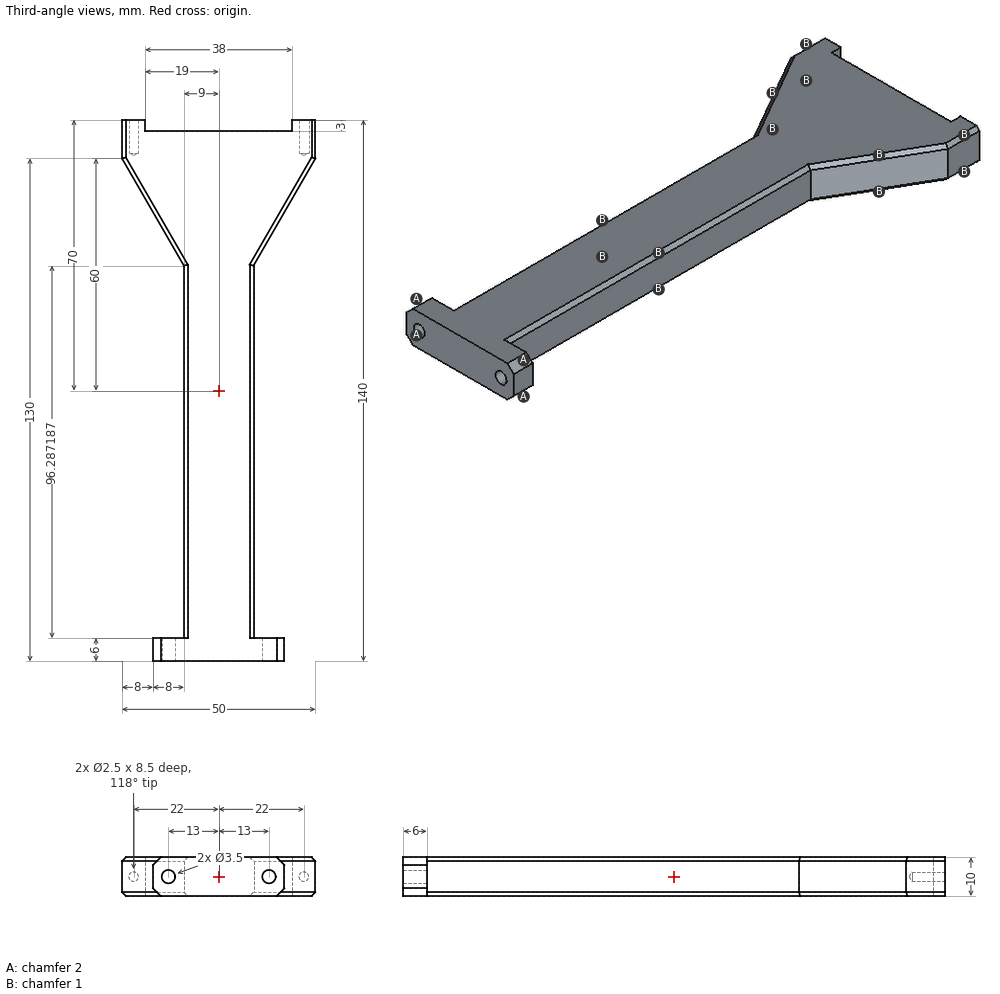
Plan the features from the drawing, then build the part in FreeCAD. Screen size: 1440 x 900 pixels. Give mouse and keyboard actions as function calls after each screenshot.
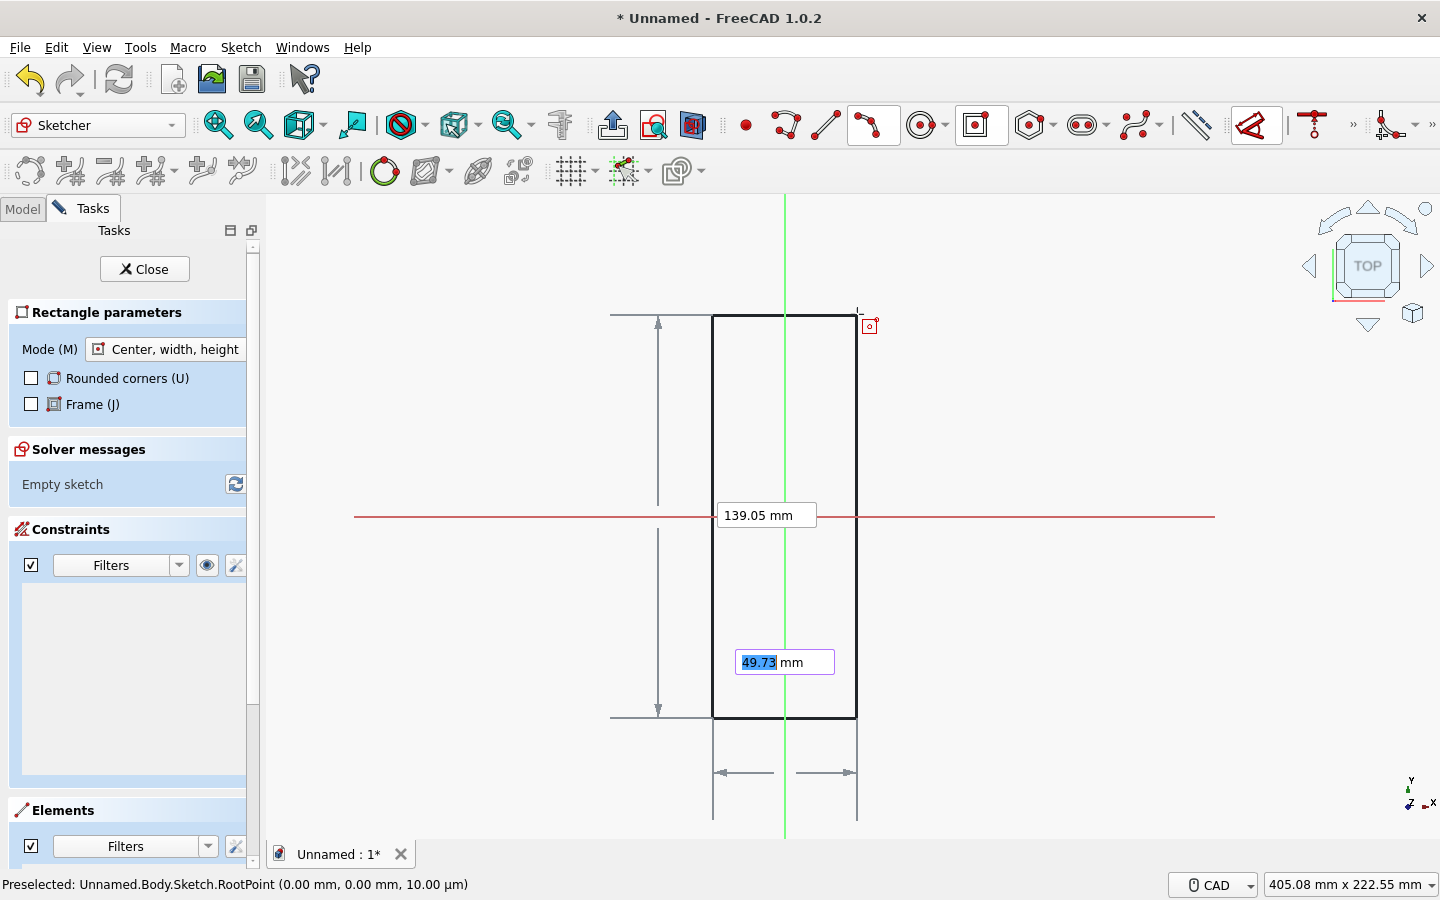
text(50)
key(Tab)
text(140)
key(Return)
key(Escape)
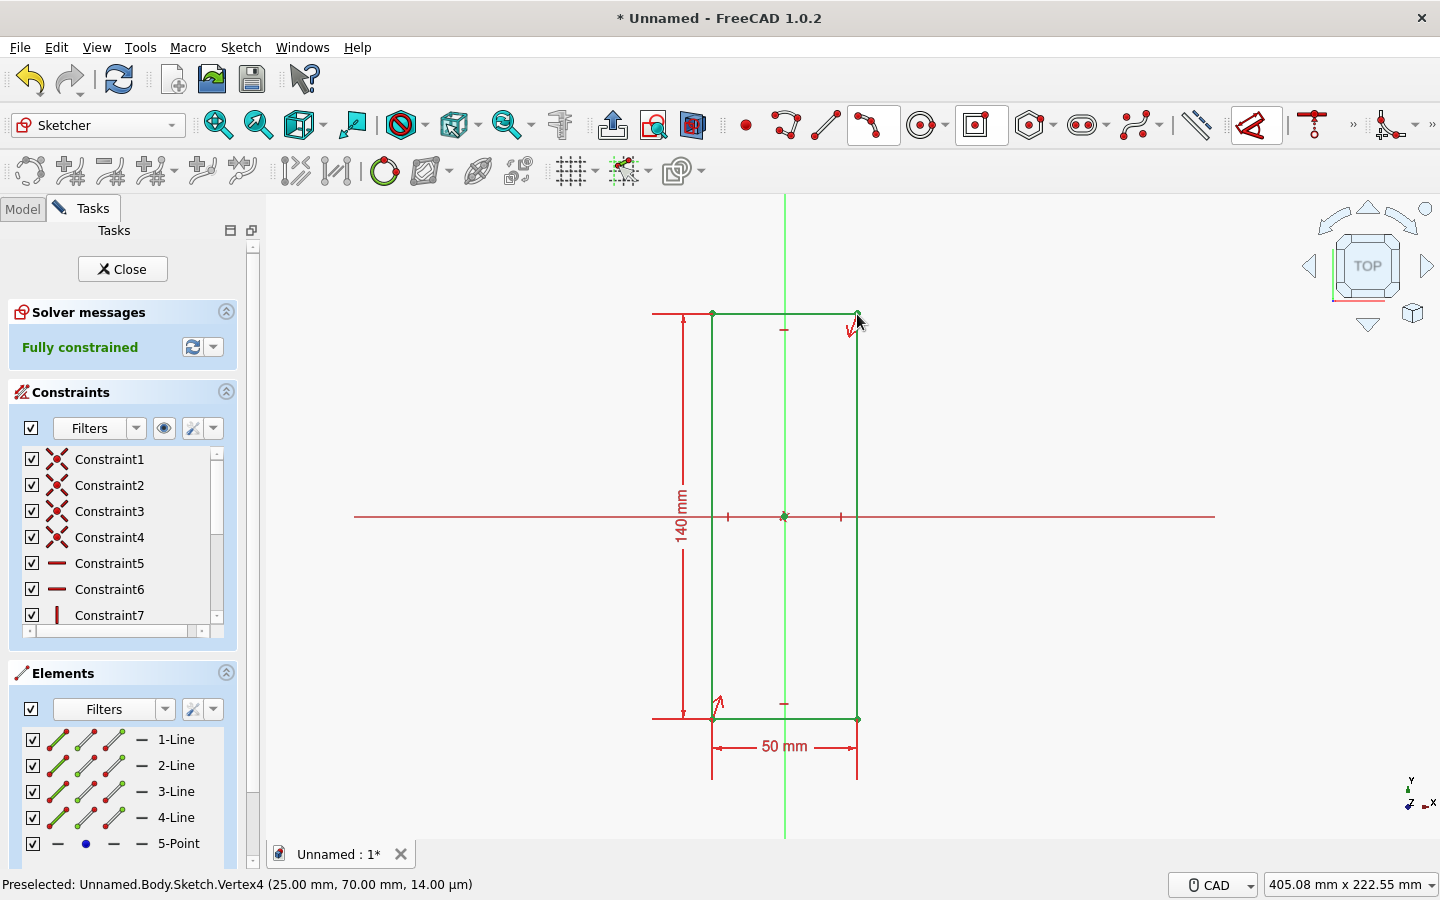
click(123, 269)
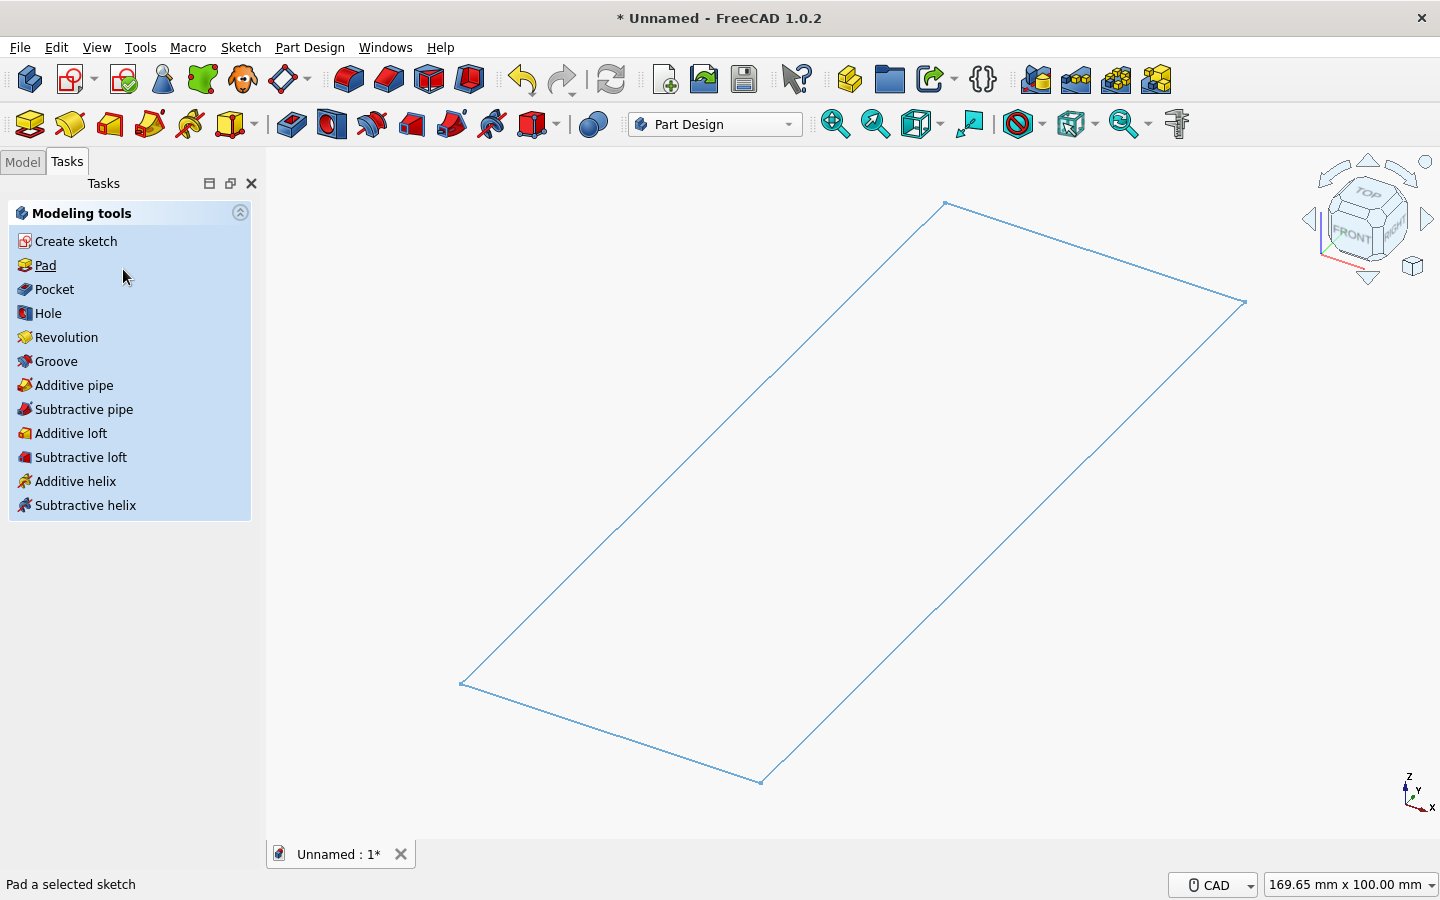
click(30, 124)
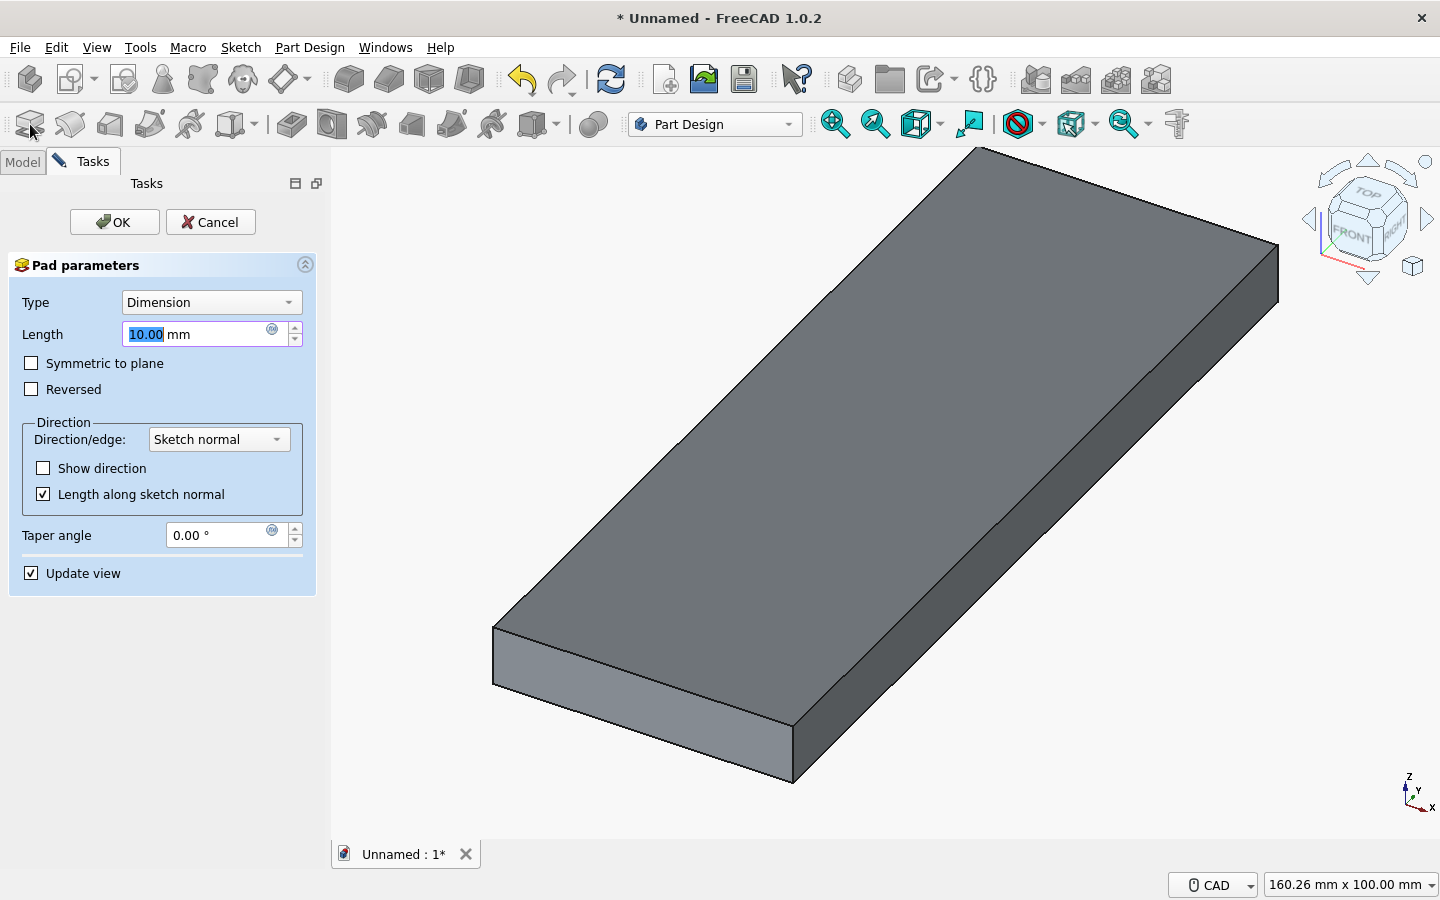
text(10)
key(Tab)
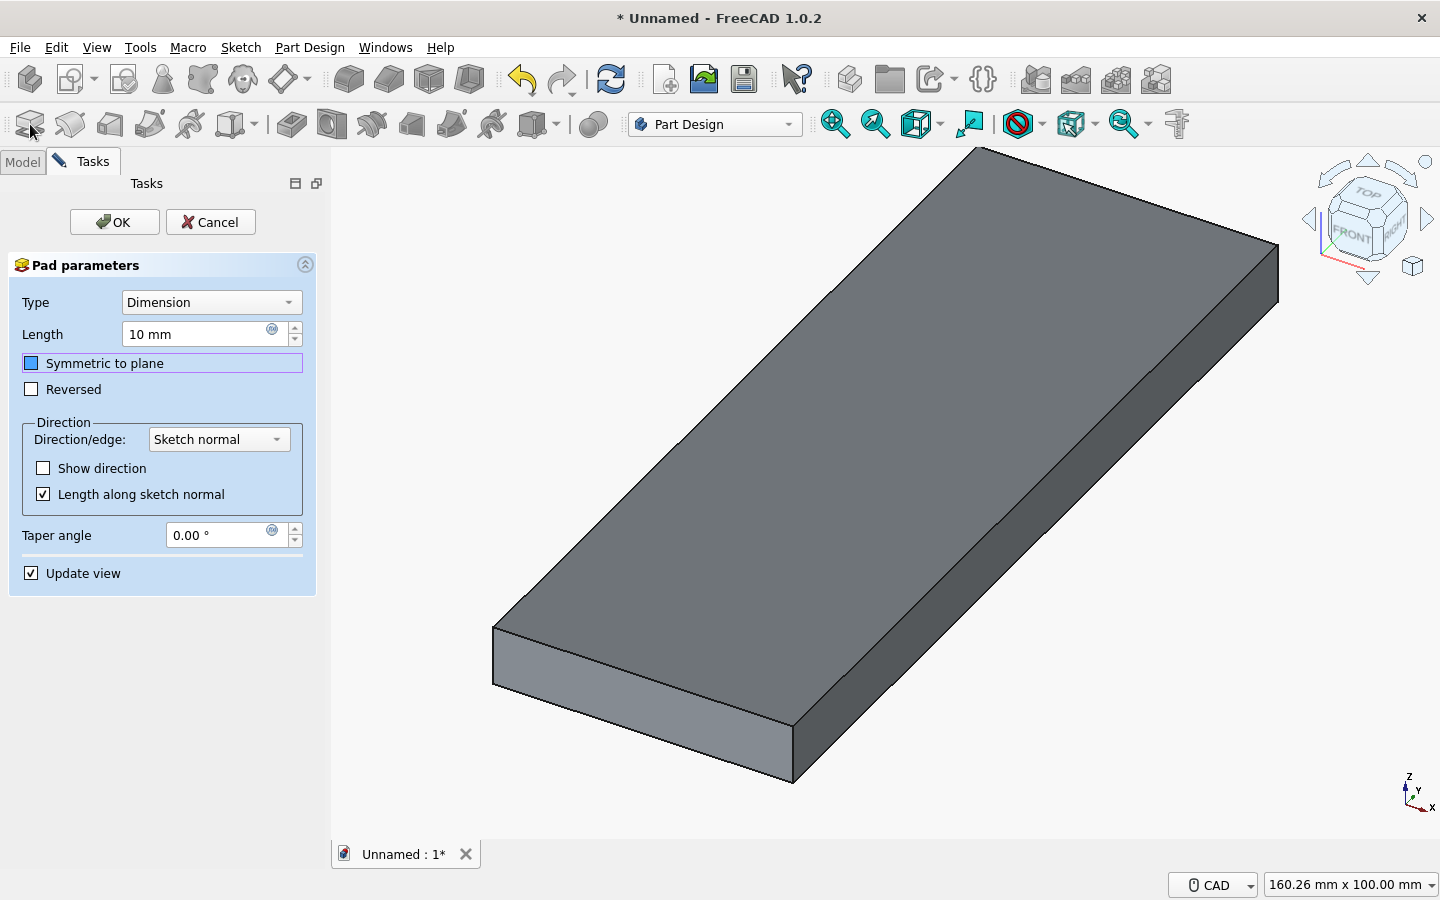
click(30, 363)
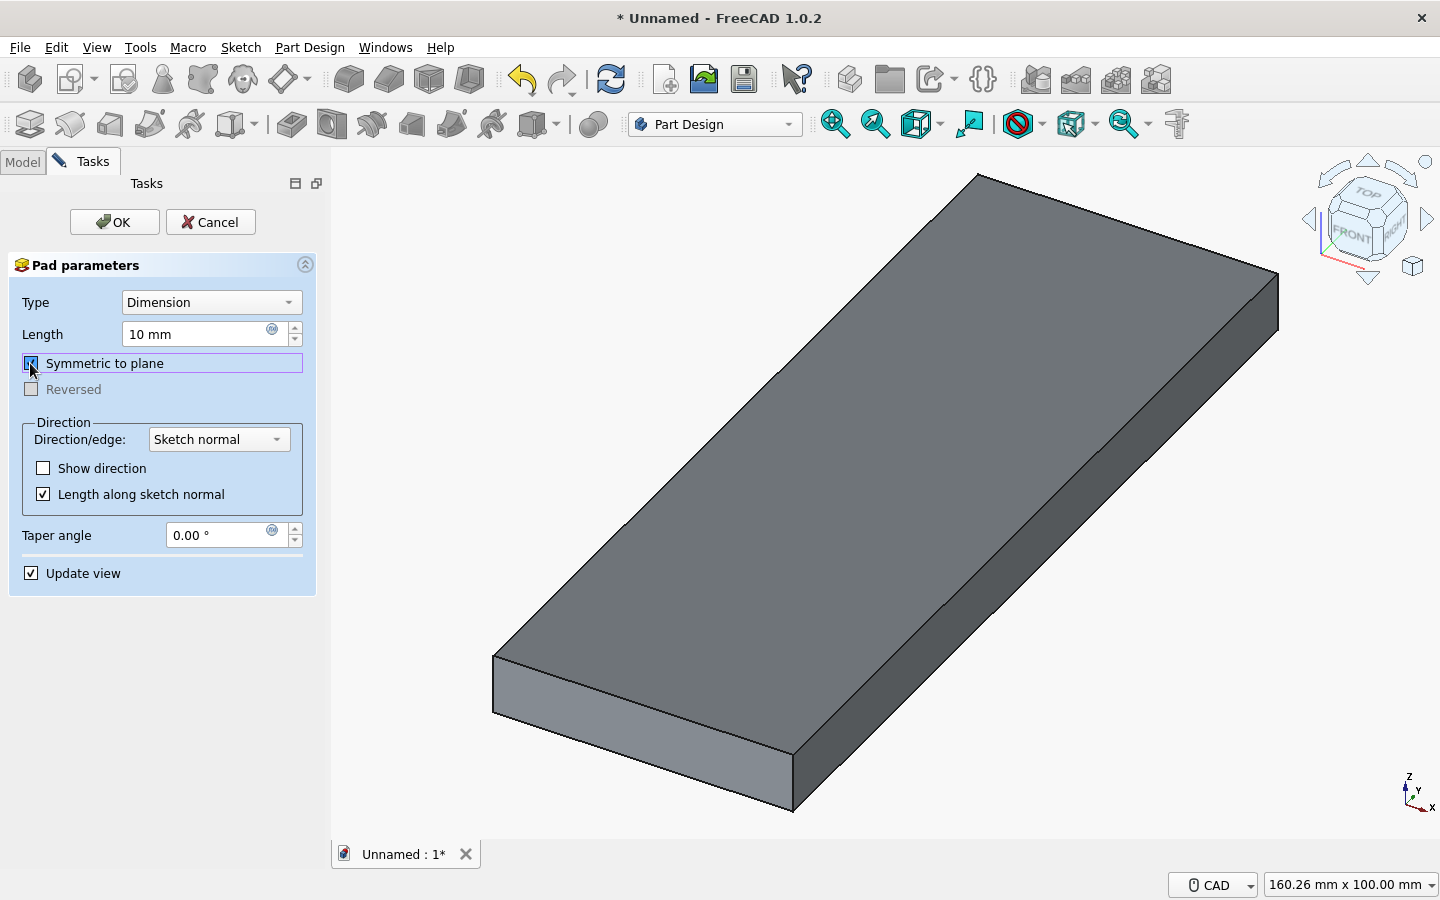
click(115, 222)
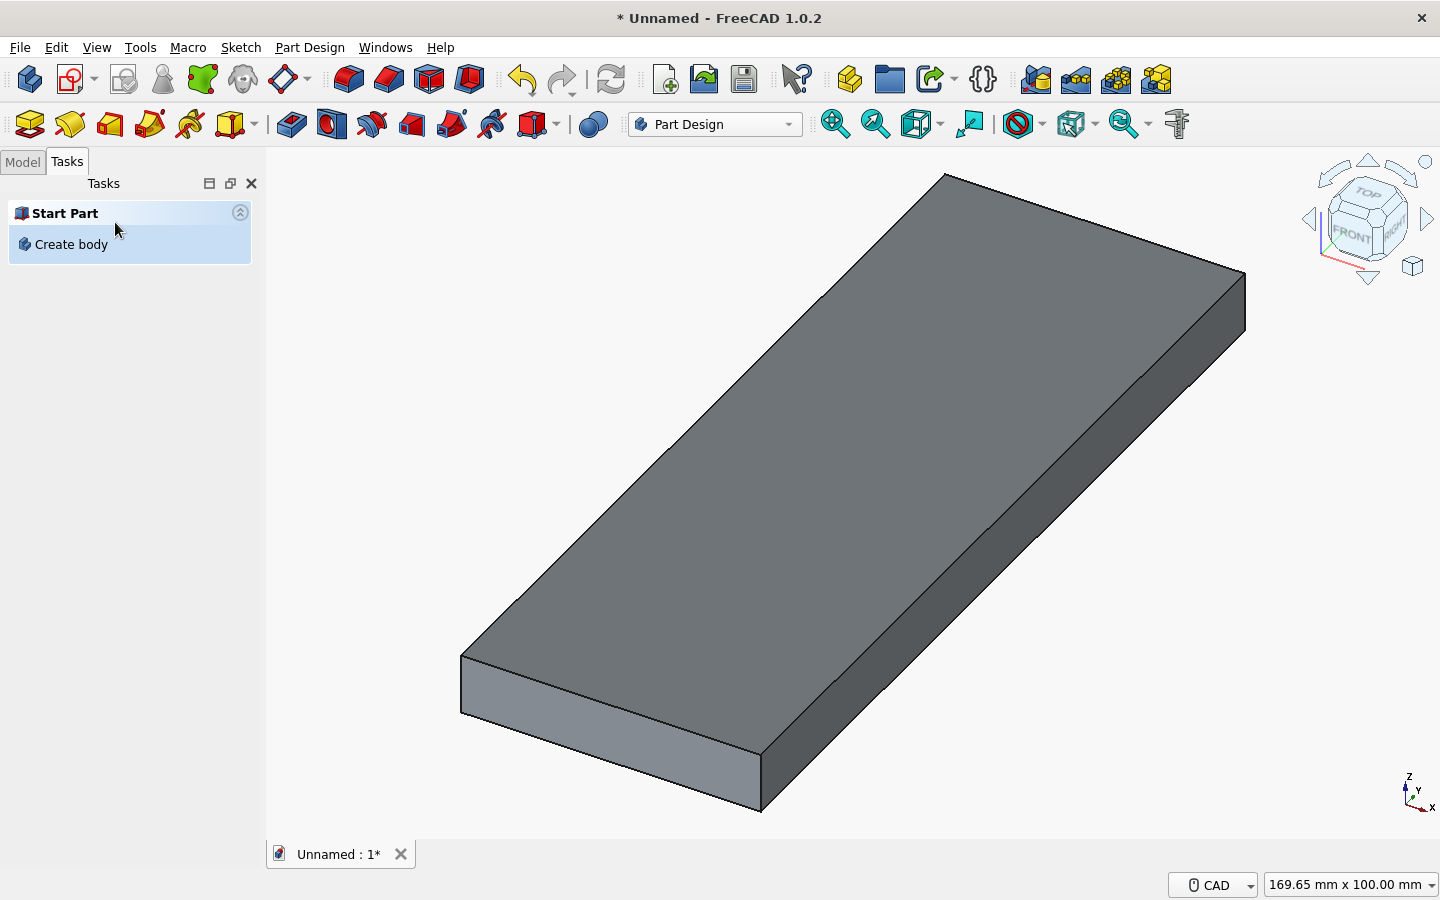
click(991, 326)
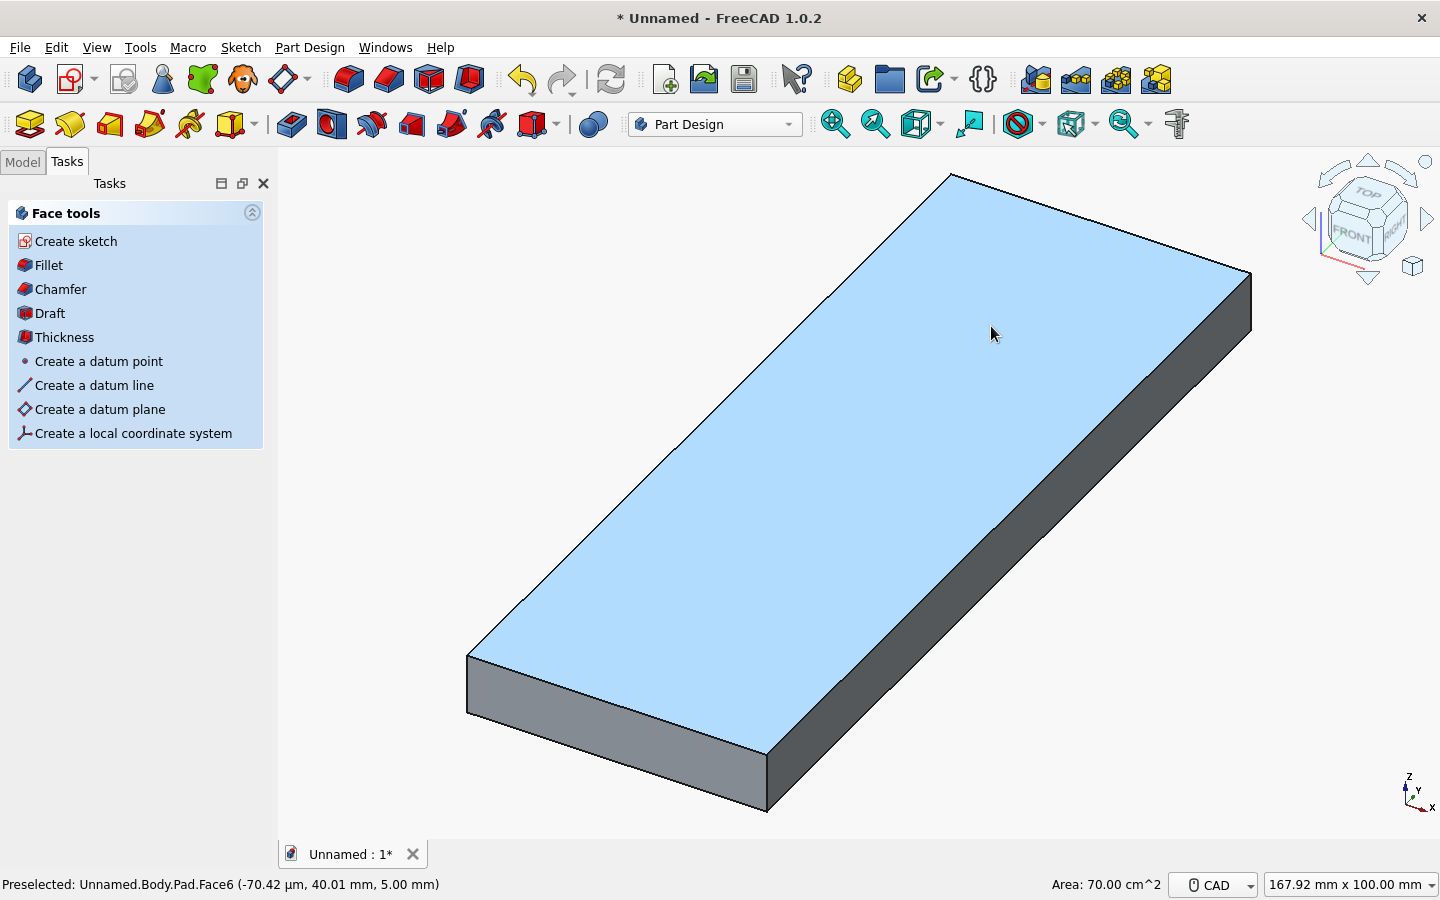
click(70, 80)